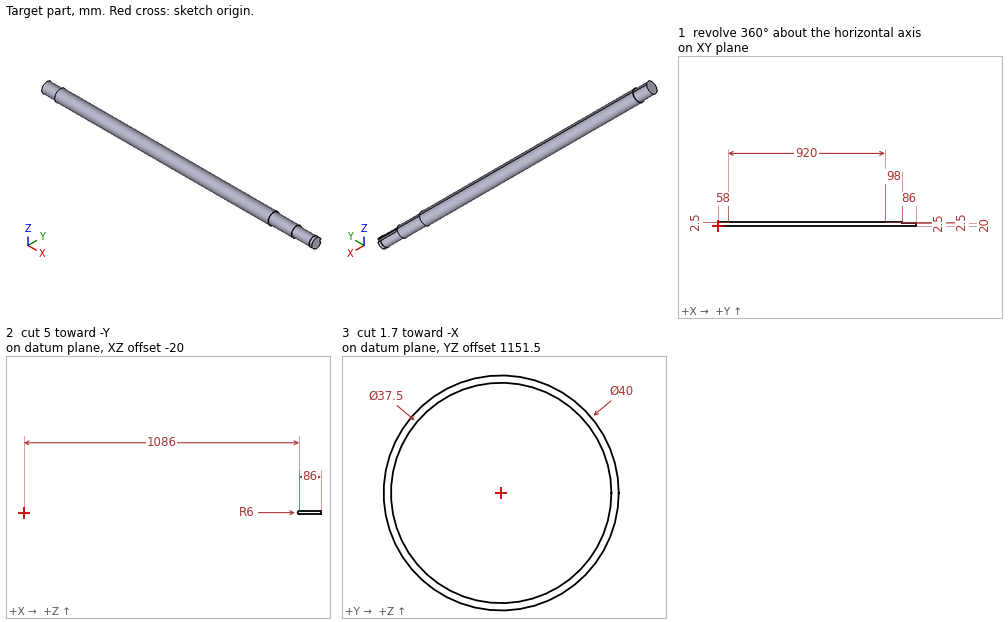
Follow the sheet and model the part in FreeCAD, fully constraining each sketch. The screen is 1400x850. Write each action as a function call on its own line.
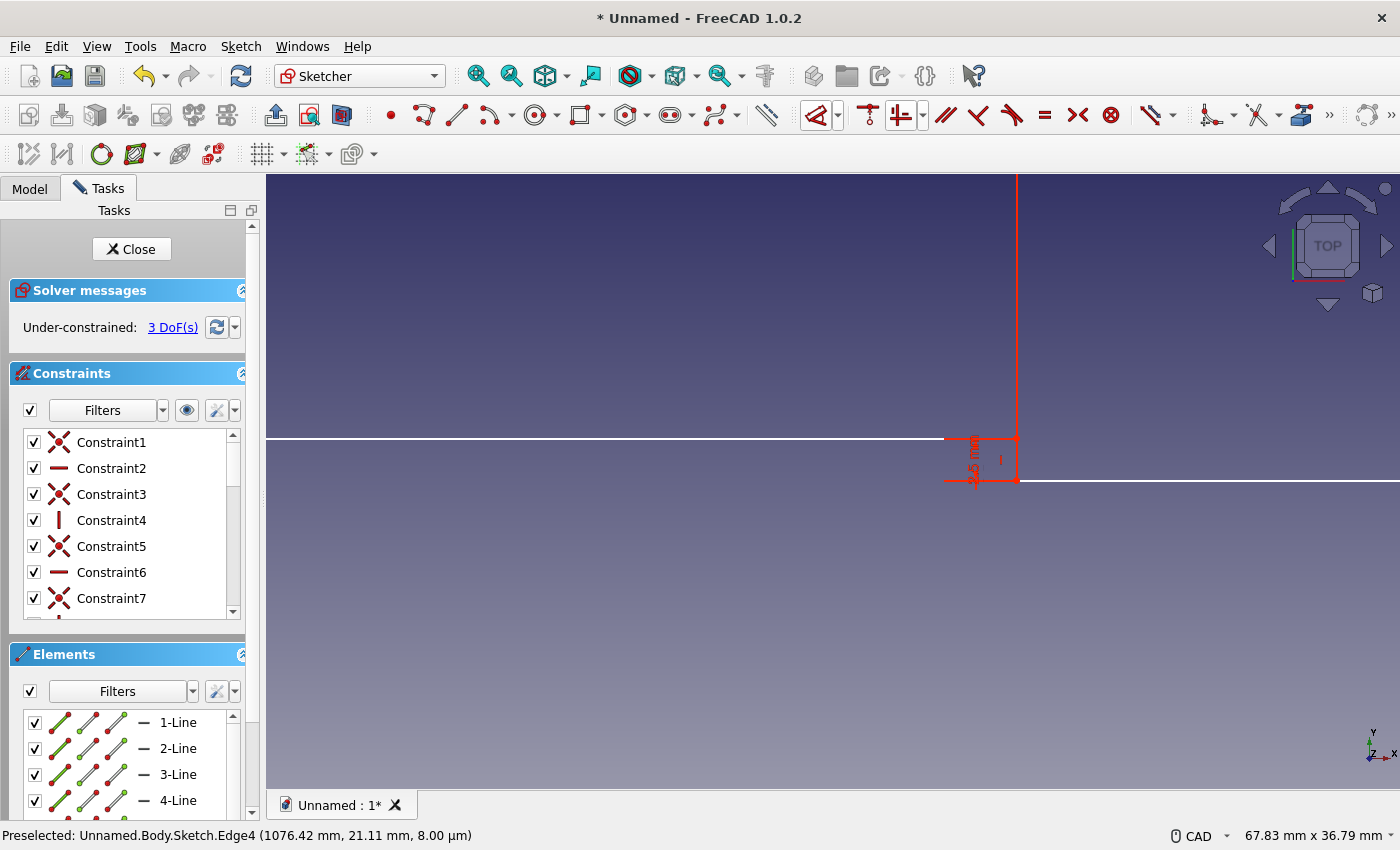
scroll(1106, 476, down, 16)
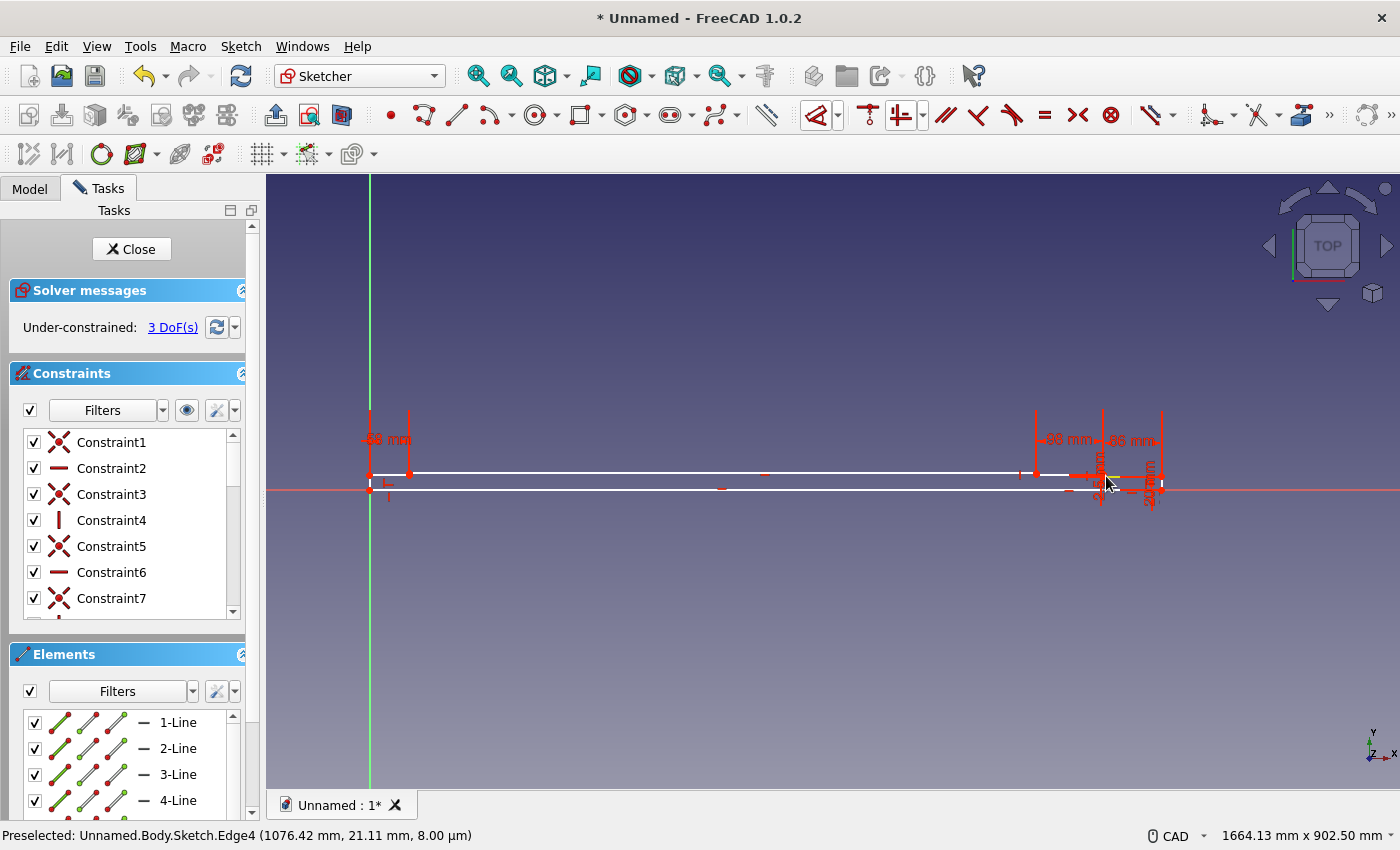
scroll(1036, 474, up, 16)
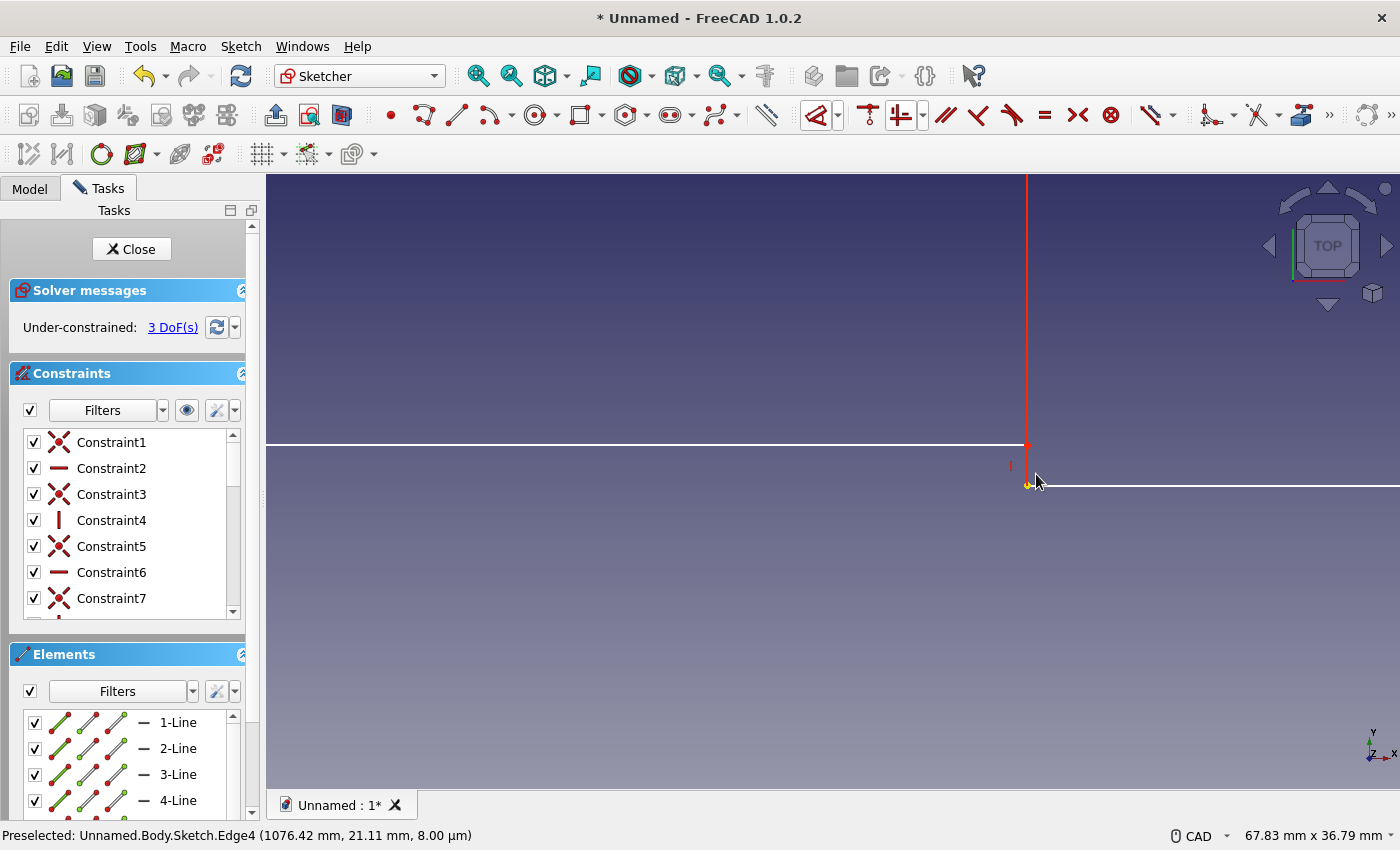
click(1027, 474)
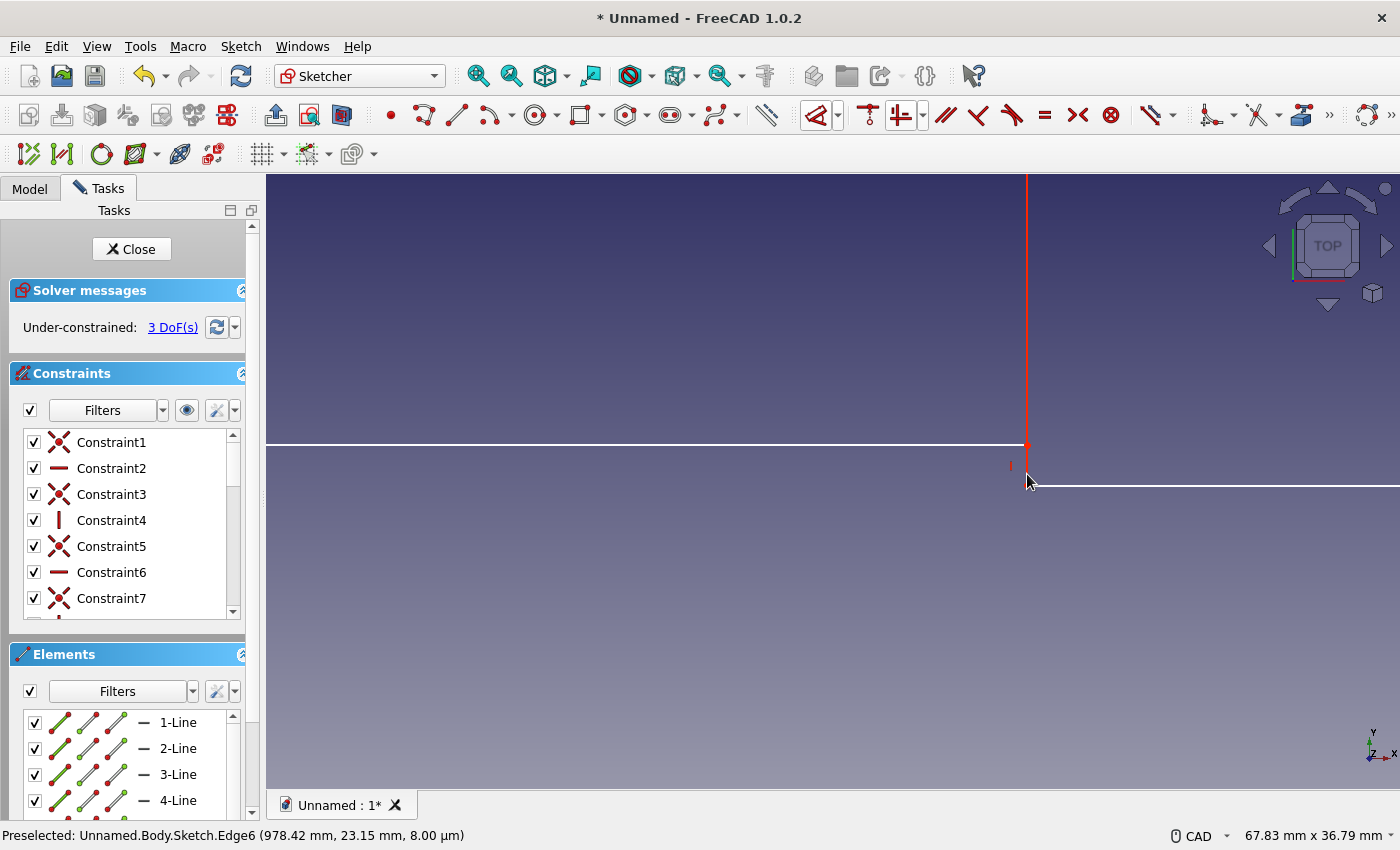
click(838, 116)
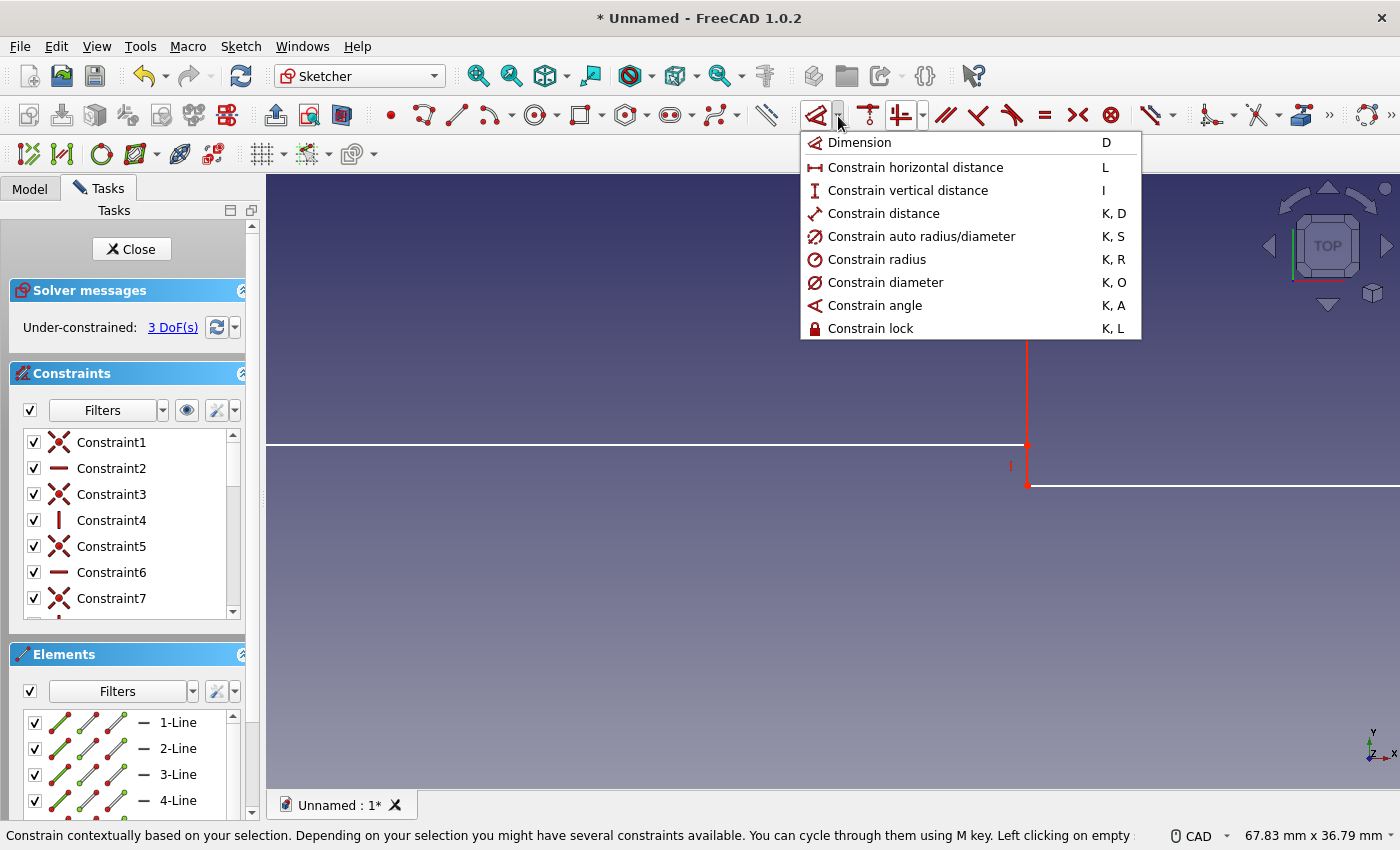
click(971, 190)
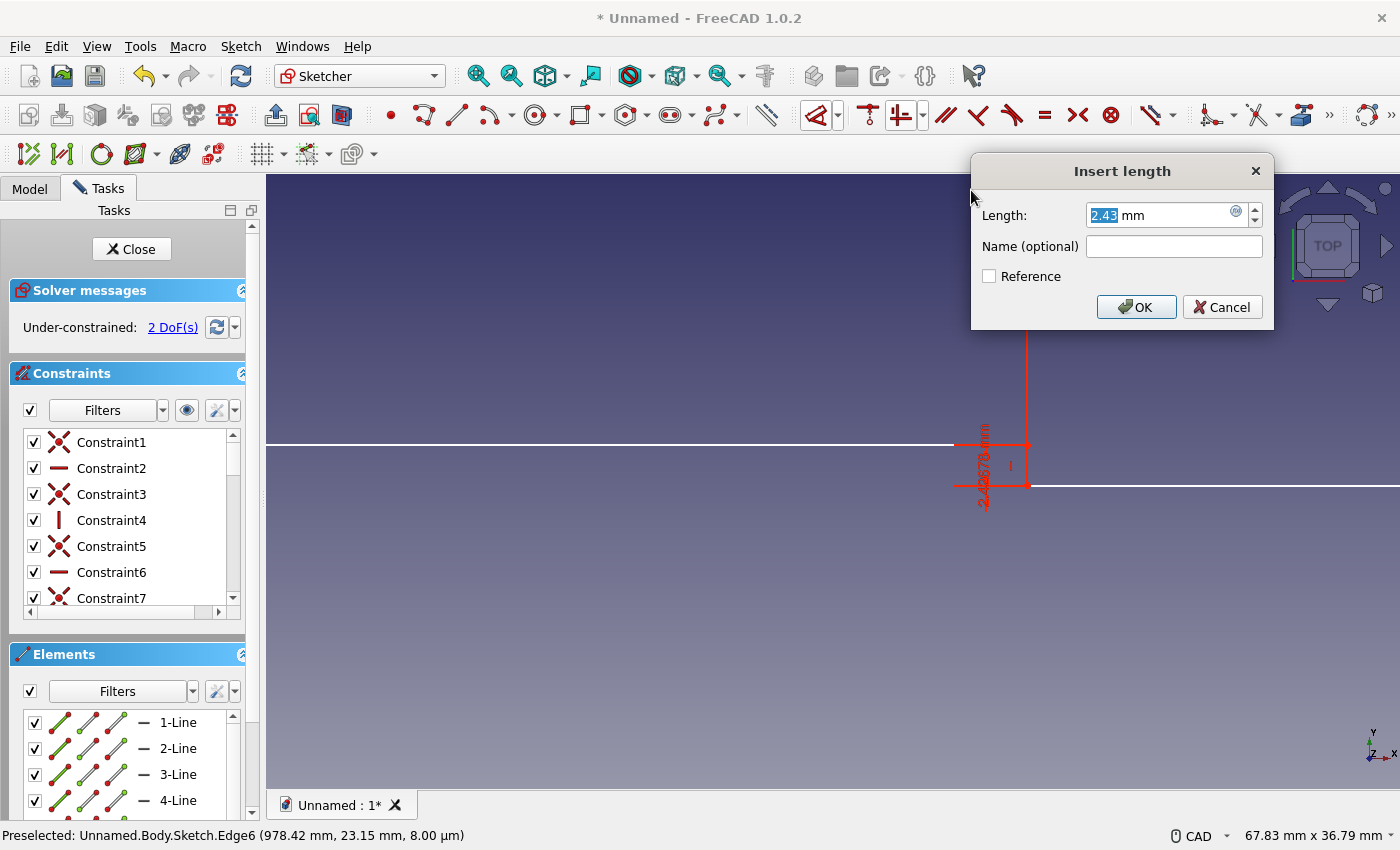
text(2.5)
key(Return)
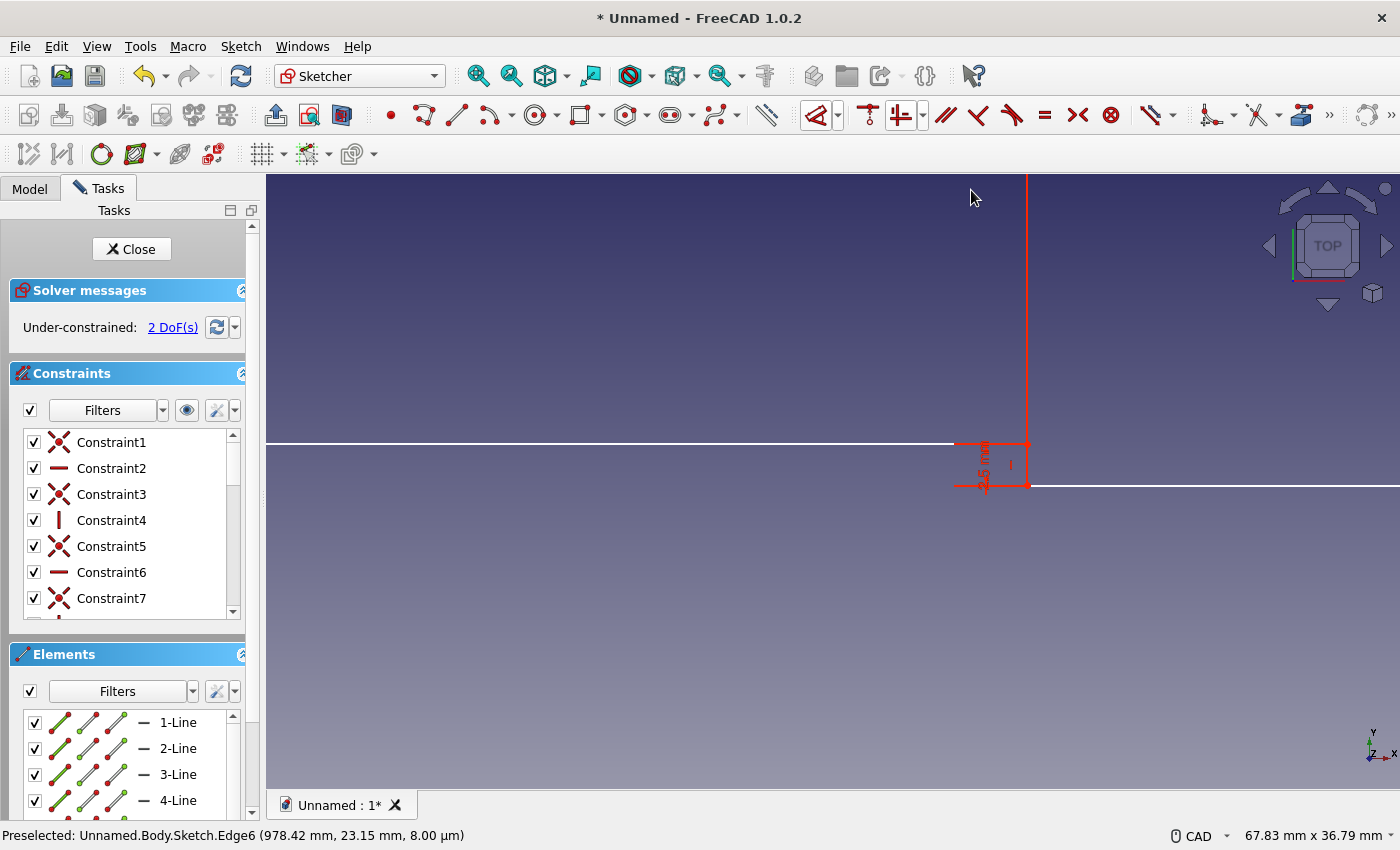
scroll(1036, 474, down, 16)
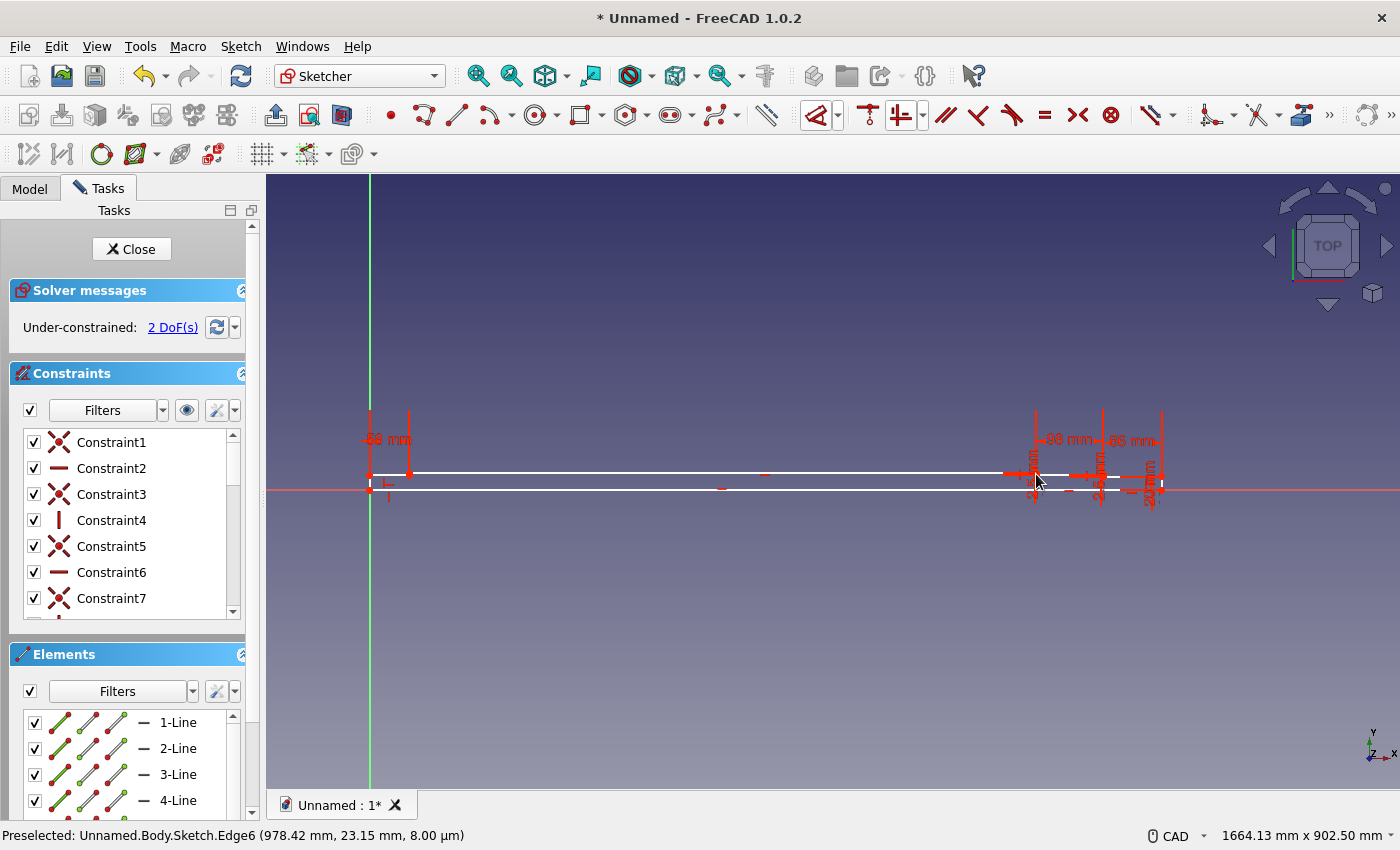
click(848, 473)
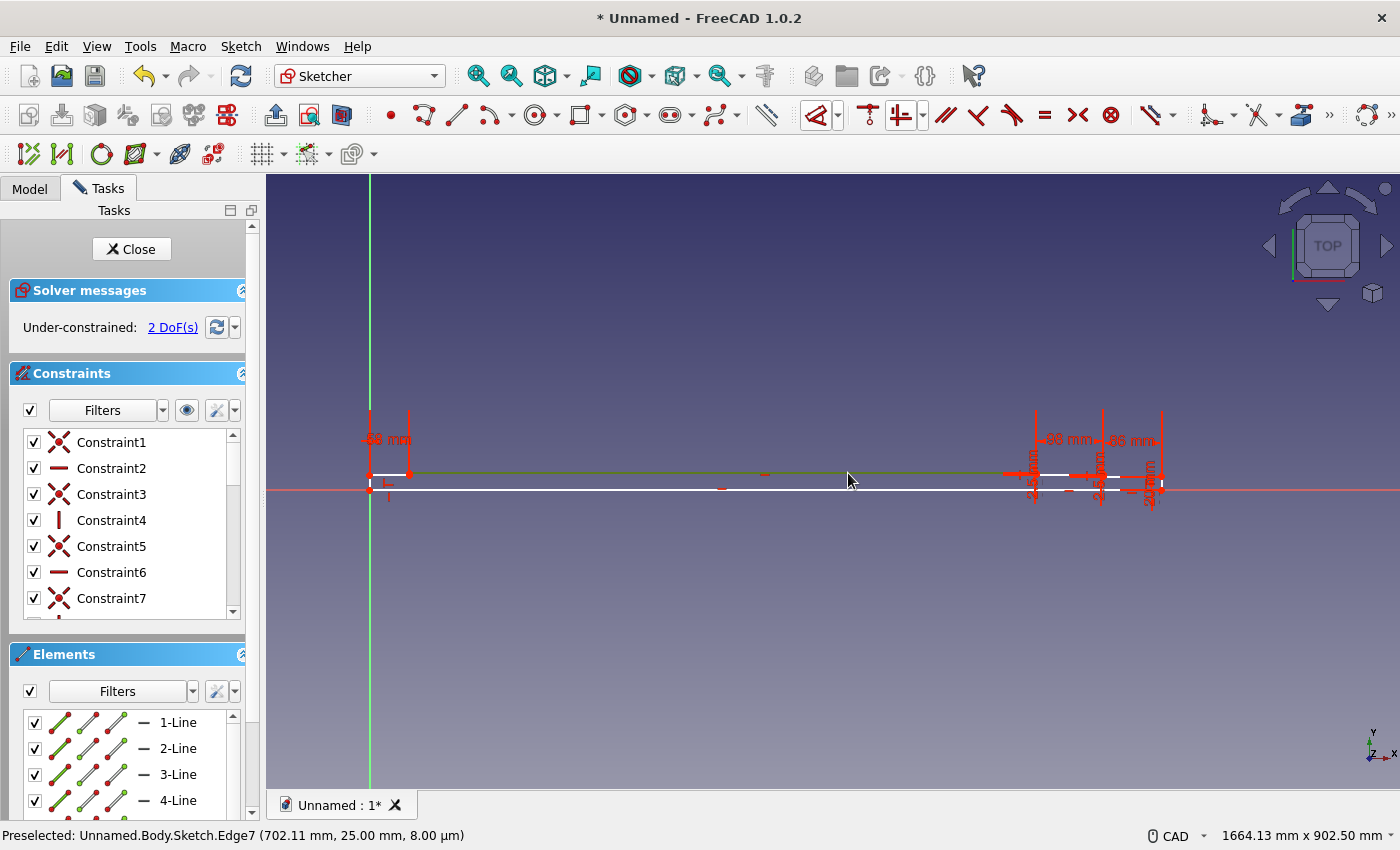
click(838, 116)